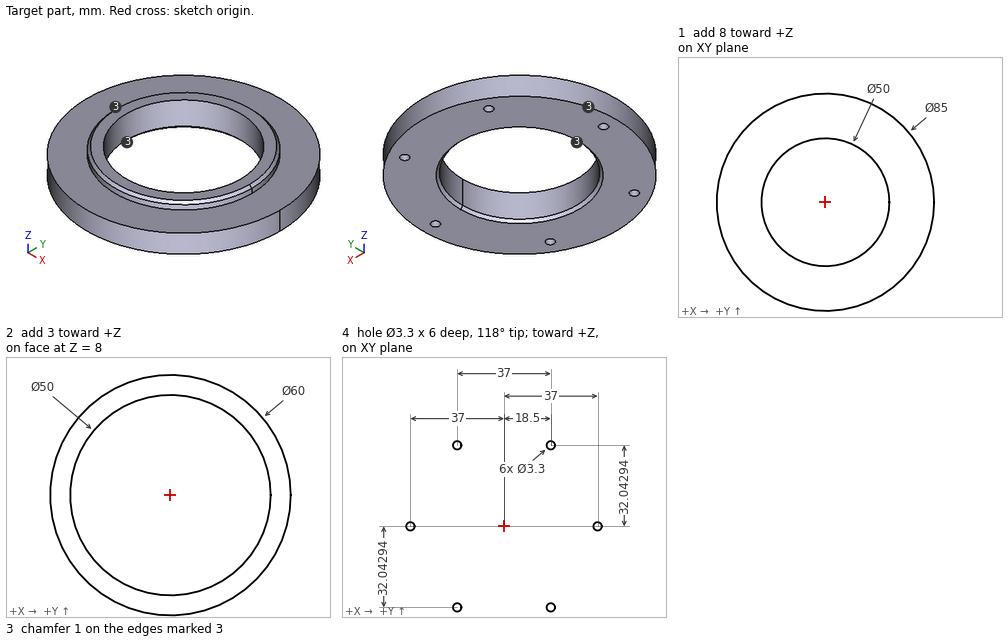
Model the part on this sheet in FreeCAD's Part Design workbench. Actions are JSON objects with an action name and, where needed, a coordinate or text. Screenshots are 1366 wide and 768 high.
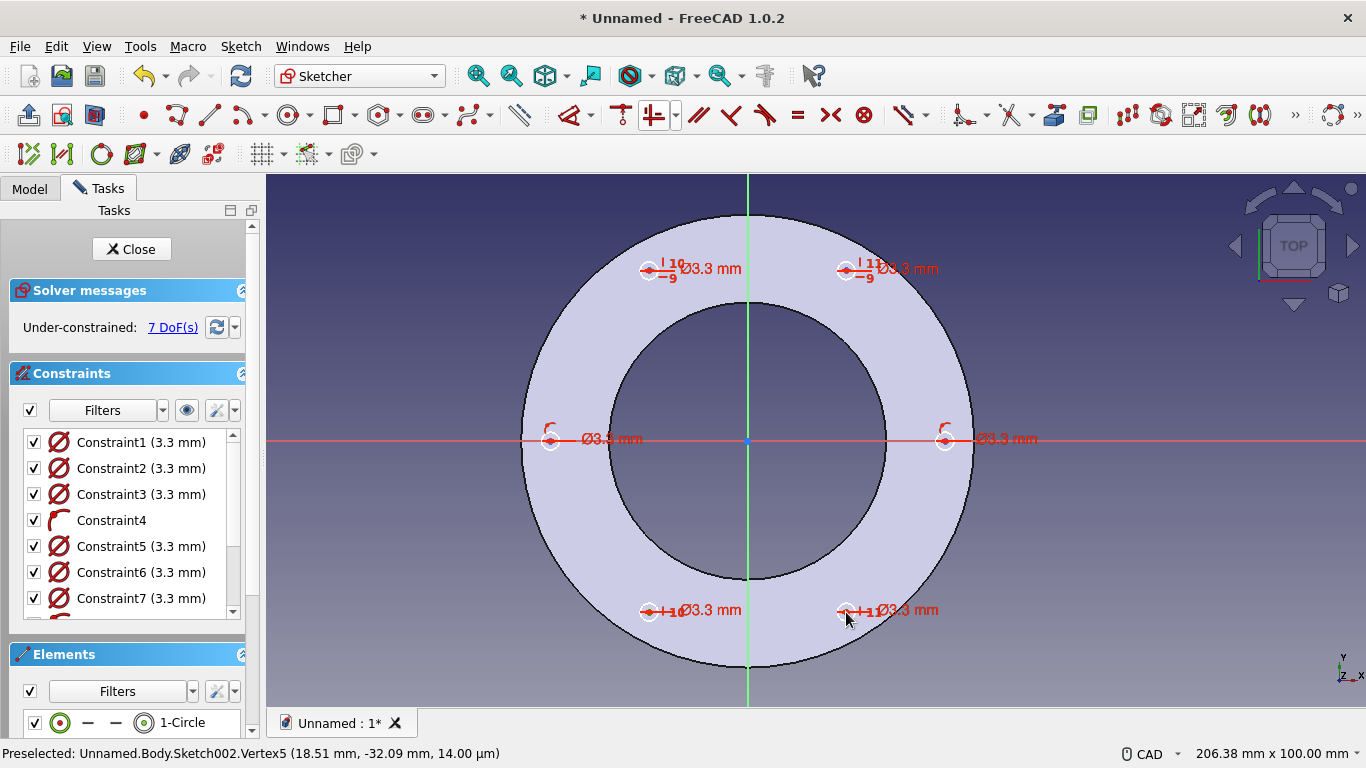
{"action": "key", "text": "h"}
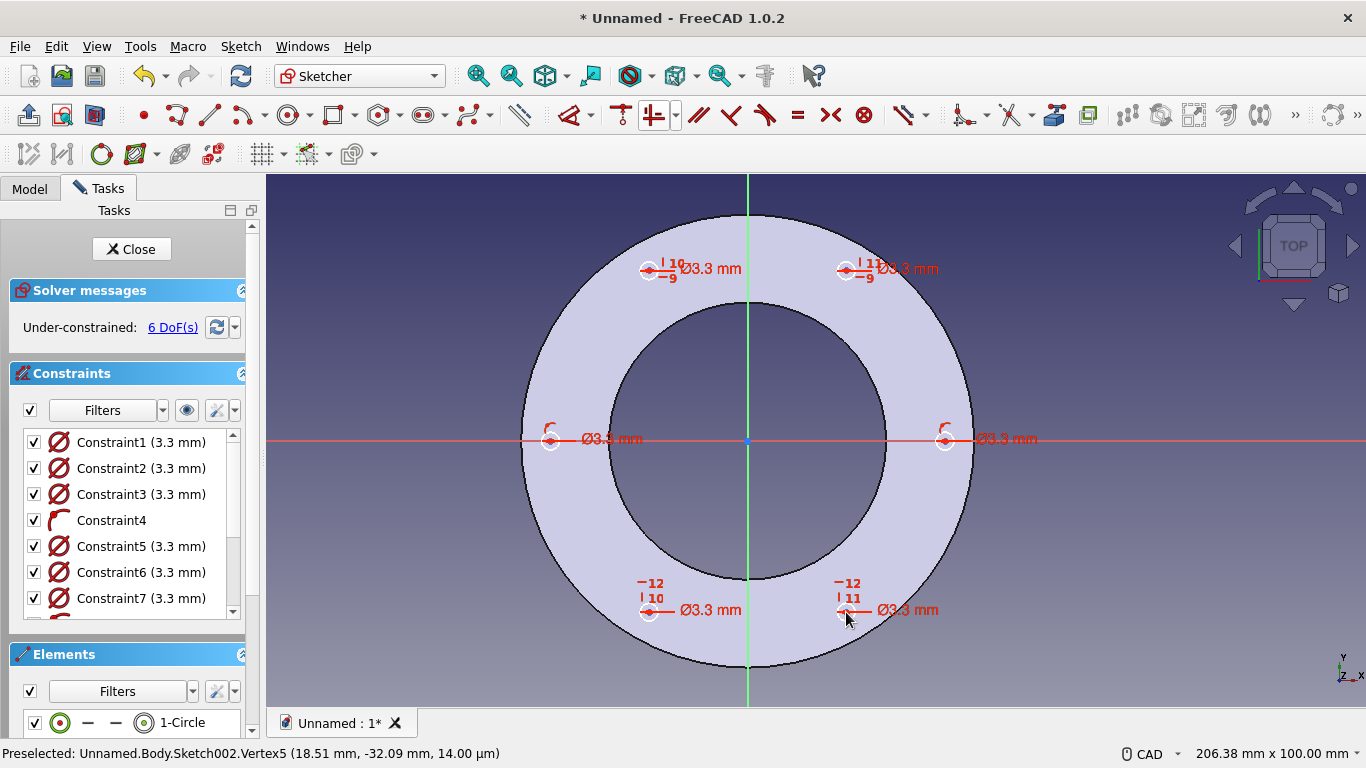
{"action": "left_click", "coordinate": [568, 116]}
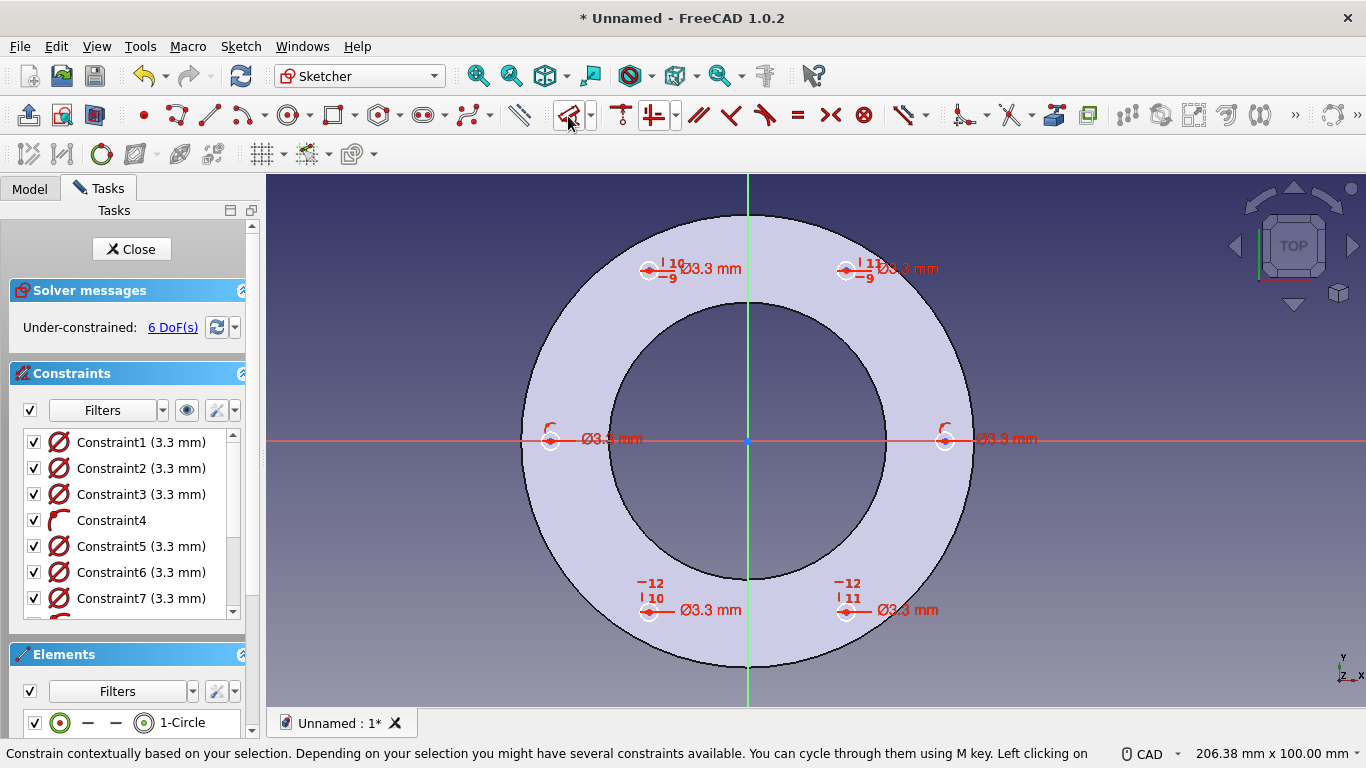
{"action": "left_click", "coordinate": [551, 441]}
{"action": "left_click", "coordinate": [649, 475]}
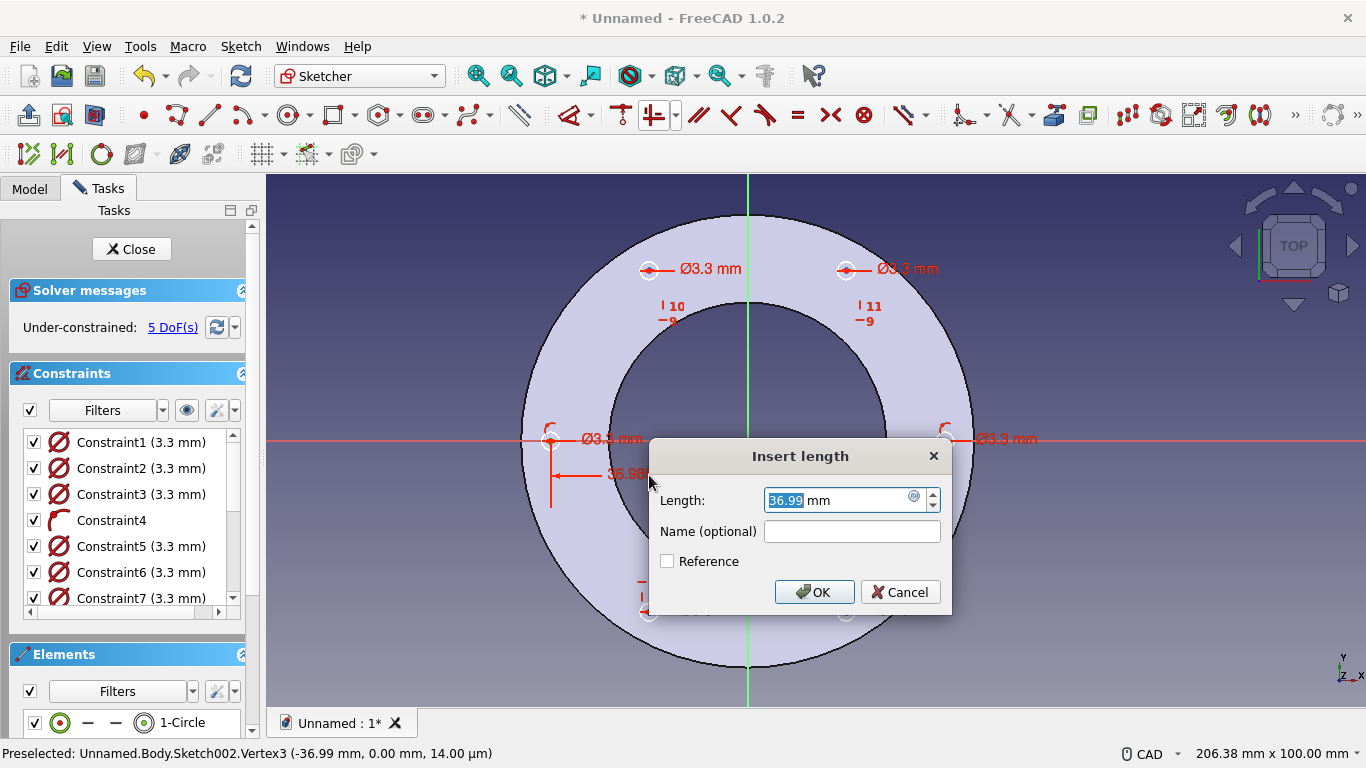
{"action": "type", "text": "37"}
{"action": "key", "text": "Return"}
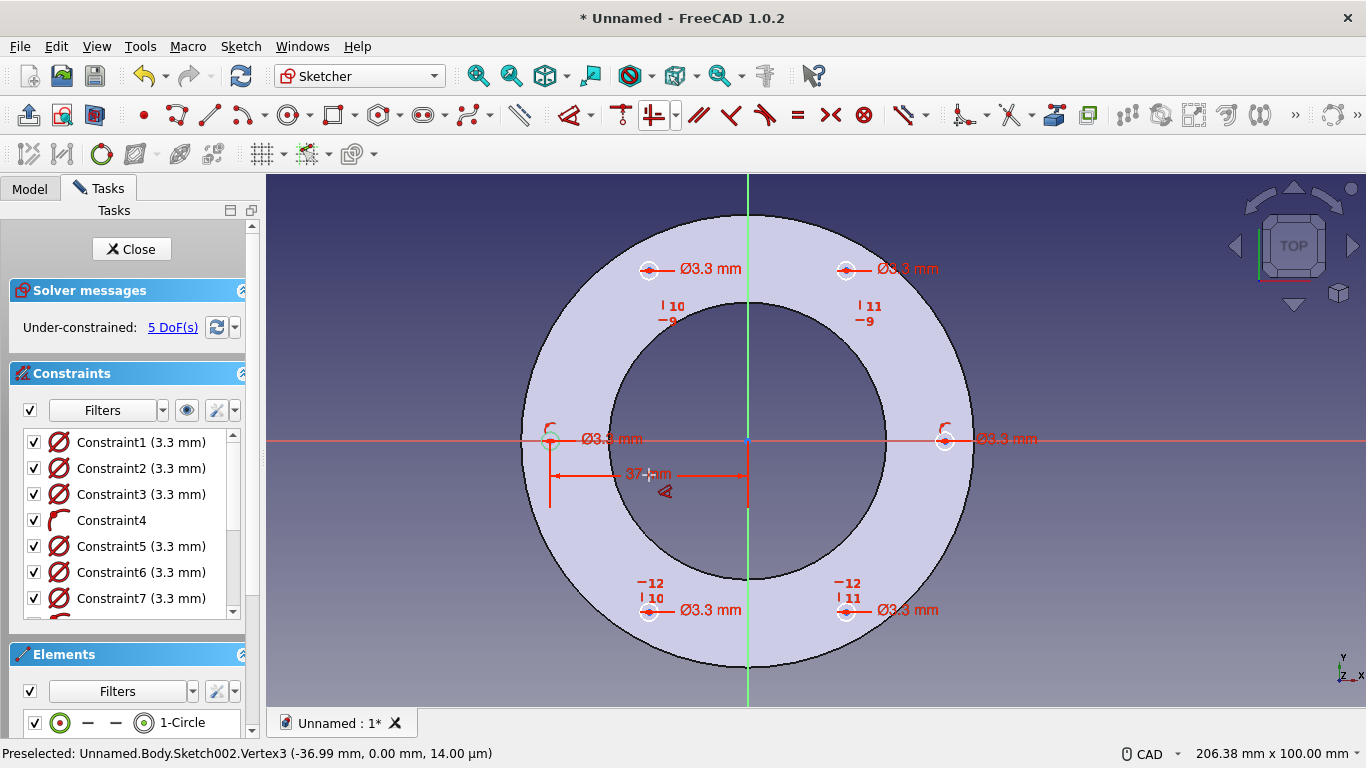
{"action": "left_click", "coordinate": [945, 441]}
{"action": "left_click", "coordinate": [846, 475]}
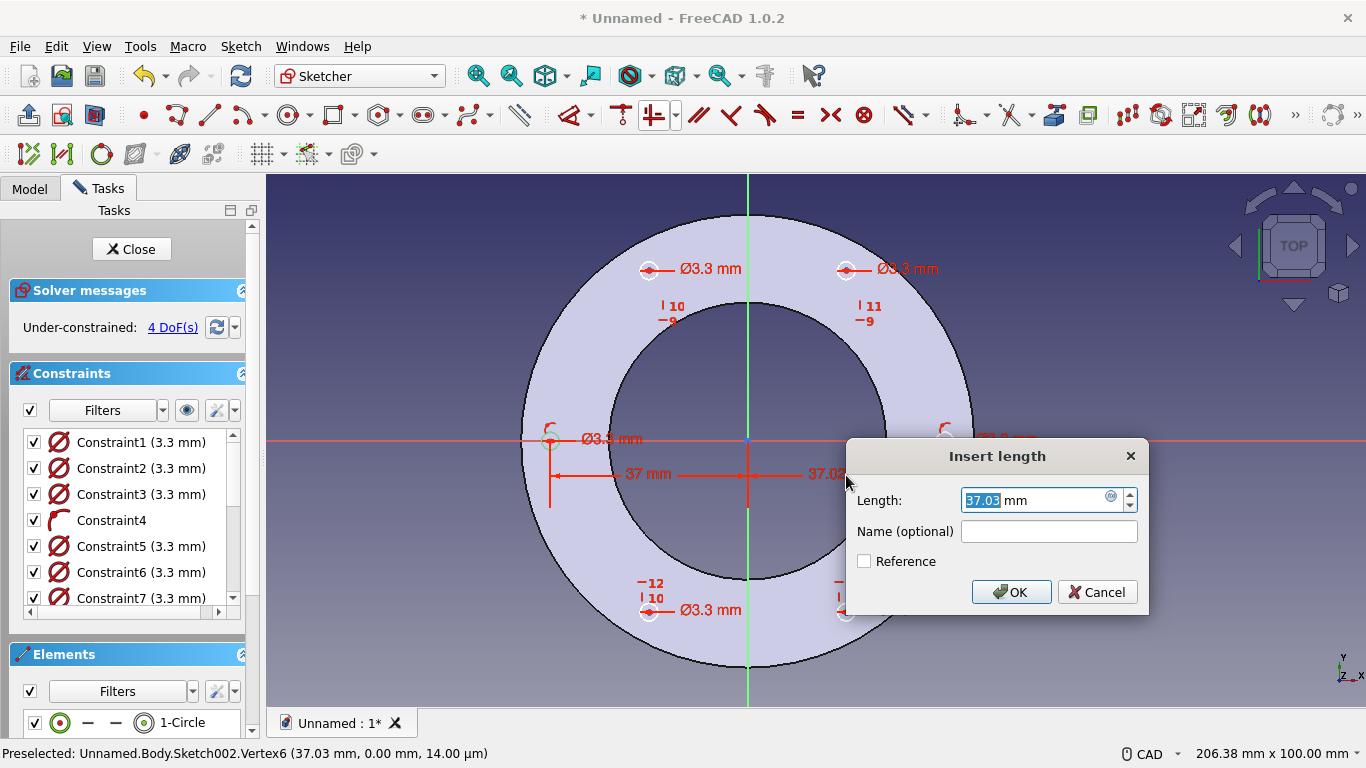
{"action": "type", "text": "37"}
{"action": "key", "text": "Return"}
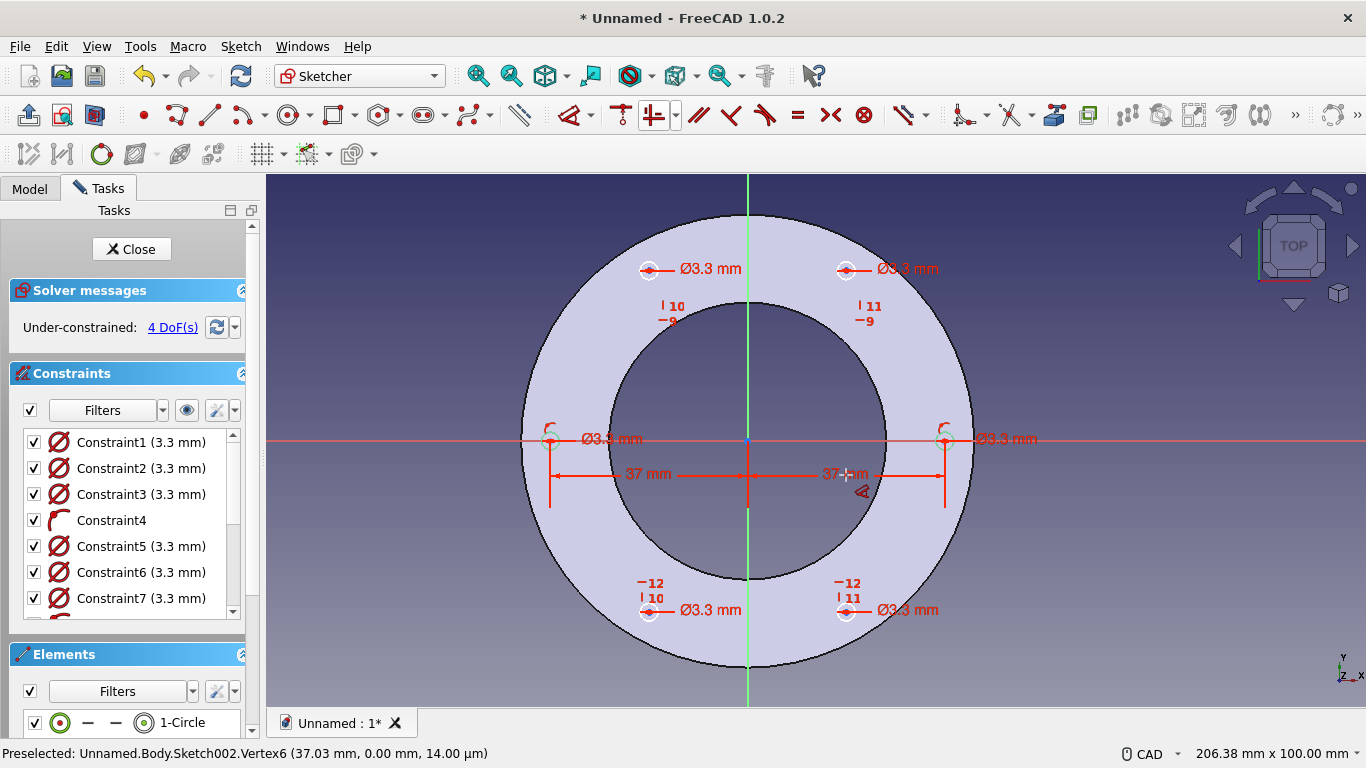
{"action": "left_click", "coordinate": [846, 271]}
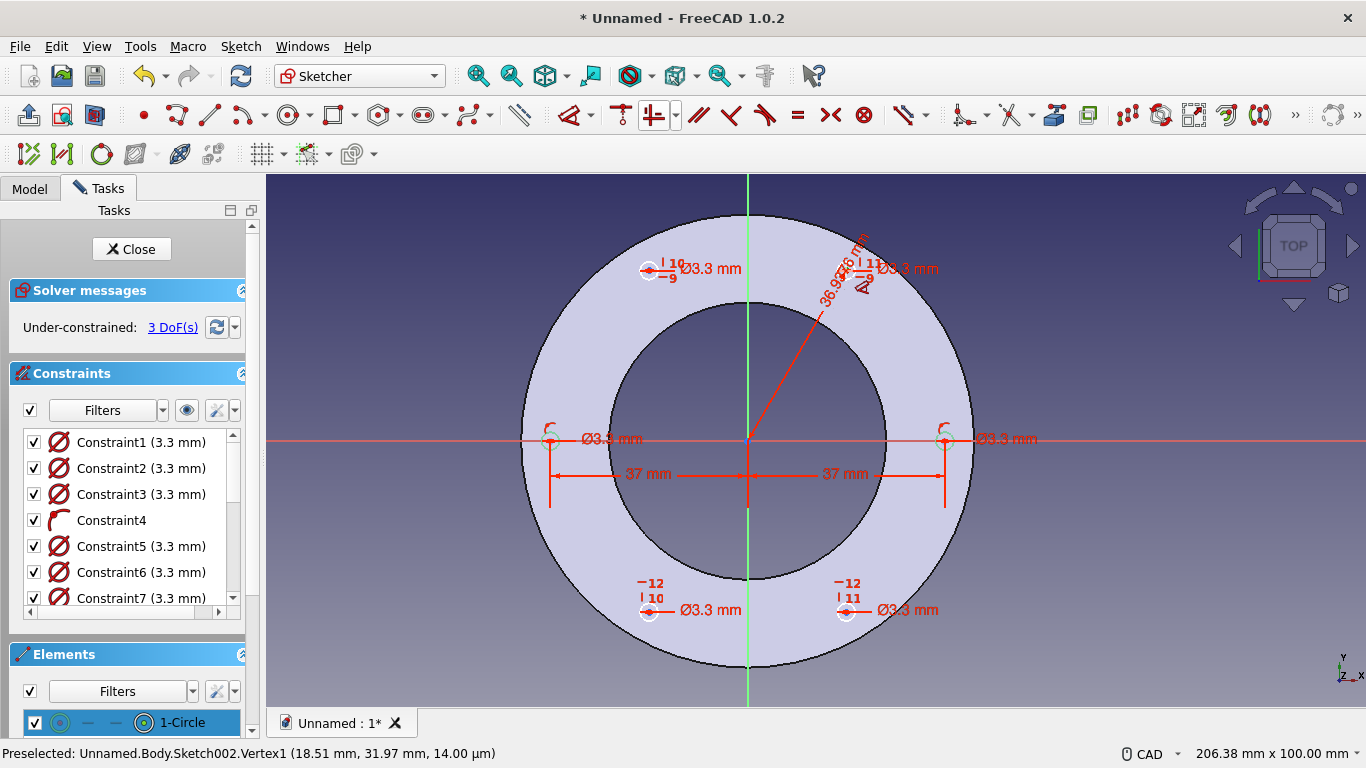
{"action": "left_click", "coordinate": [649, 271]}
{"action": "left_click", "coordinate": [702, 237]}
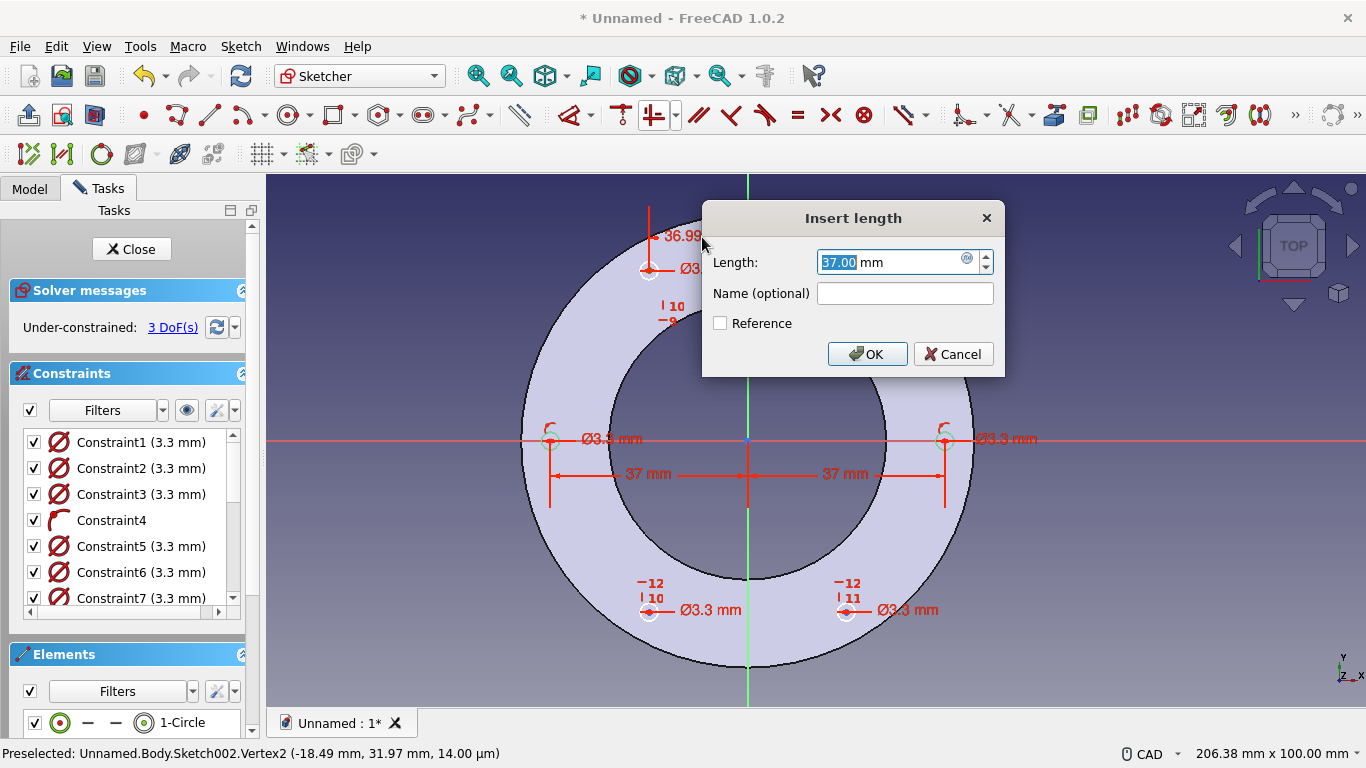
{"action": "type", "text": "37"}
{"action": "key", "text": "Return"}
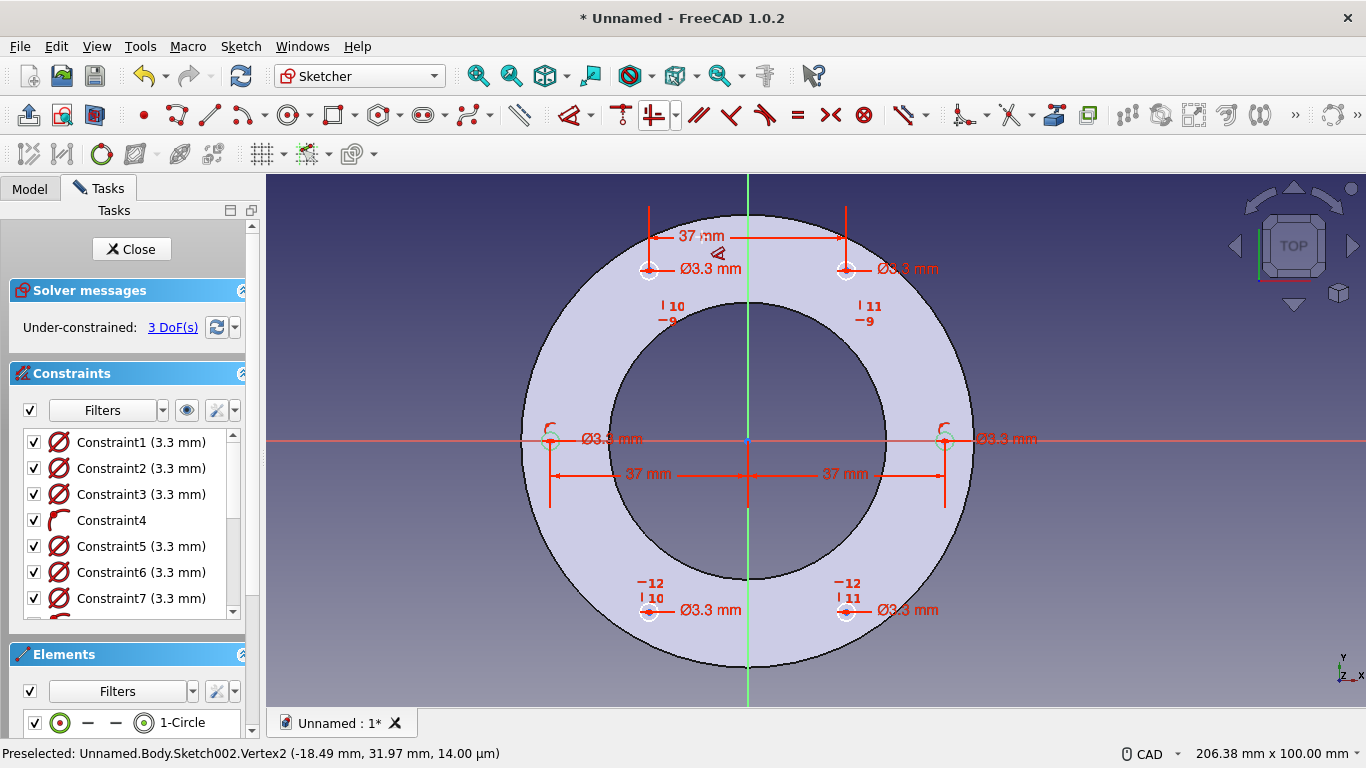
{"action": "left_click", "coordinate": [846, 271]}
{"action": "left_click", "coordinate": [797, 237]}